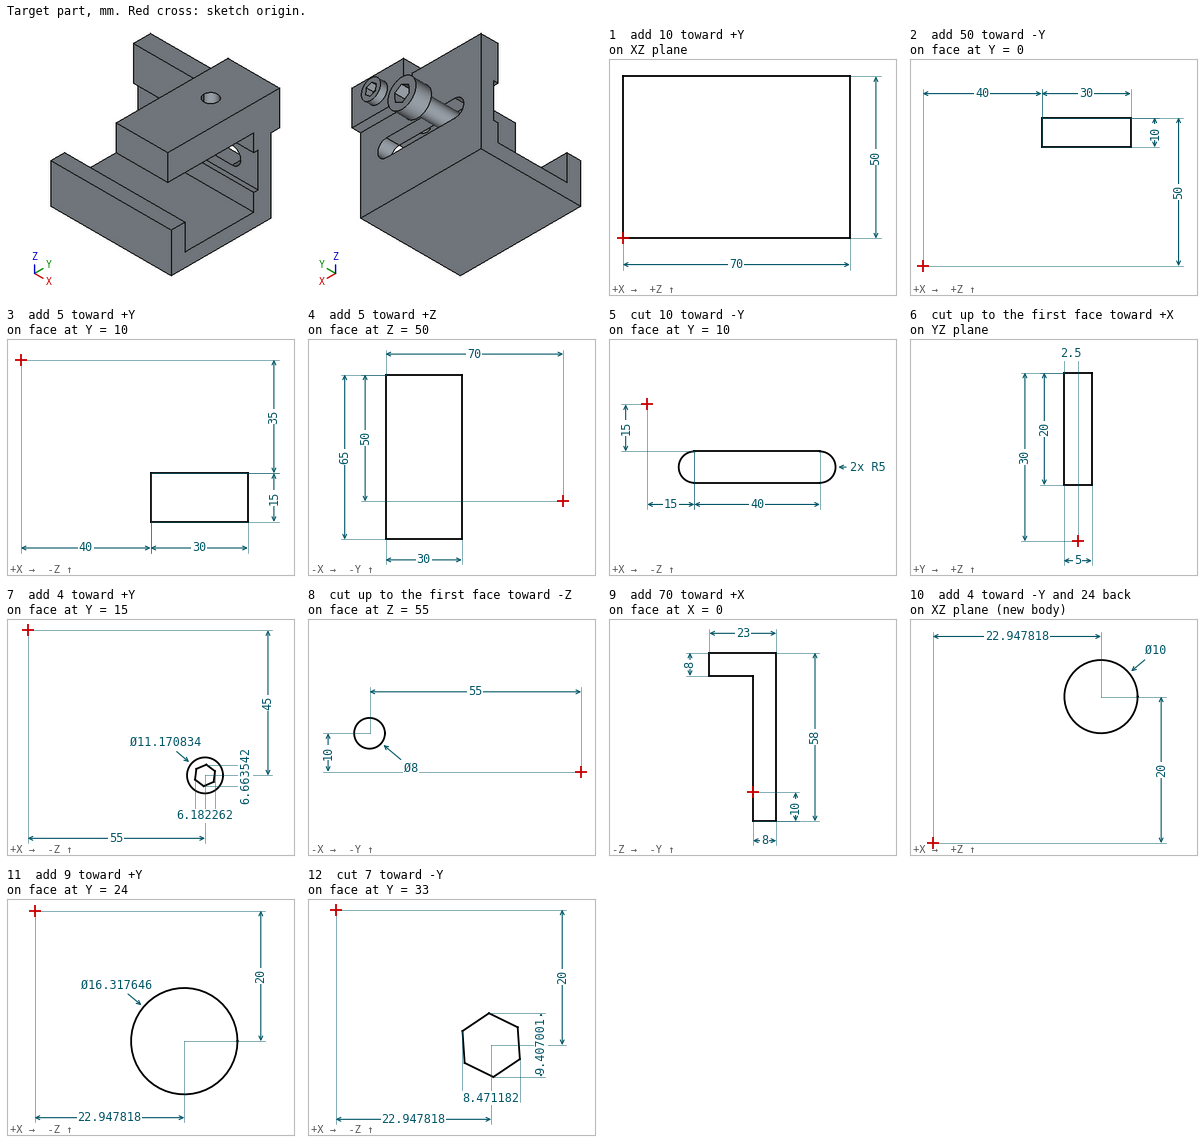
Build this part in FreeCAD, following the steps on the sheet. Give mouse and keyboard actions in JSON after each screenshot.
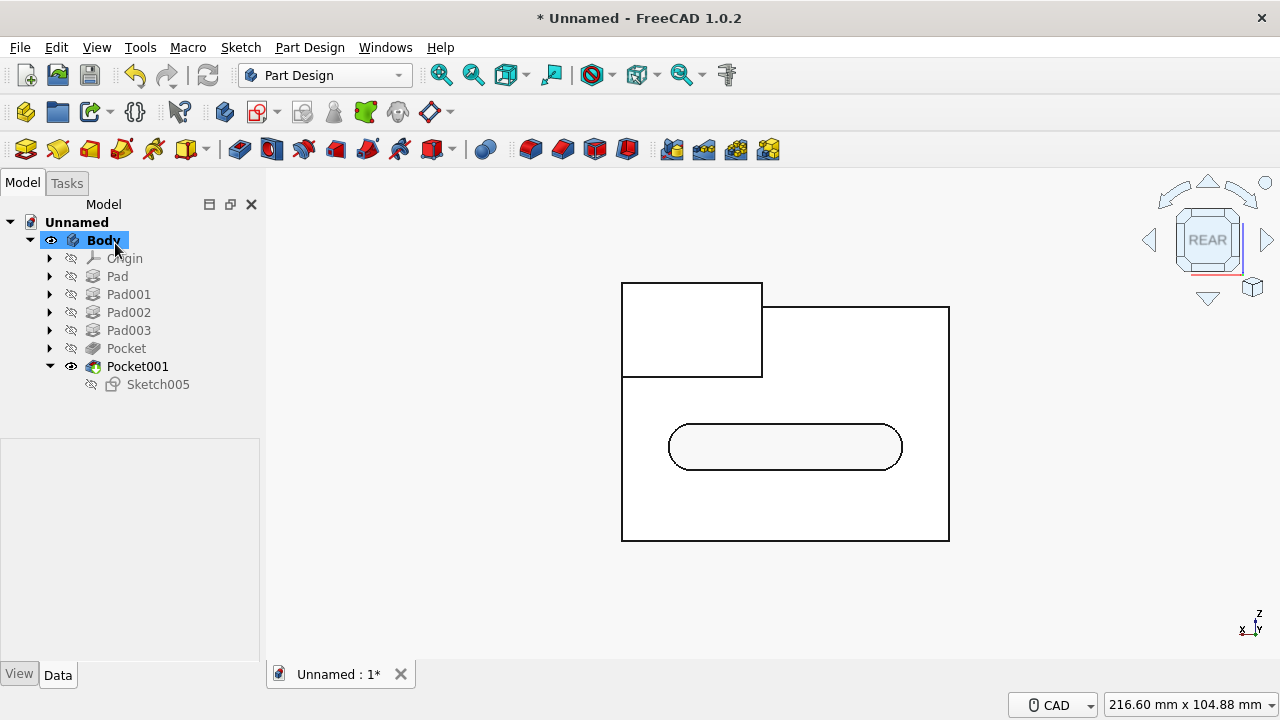
{"action": "left_click", "coordinate": [672, 329]}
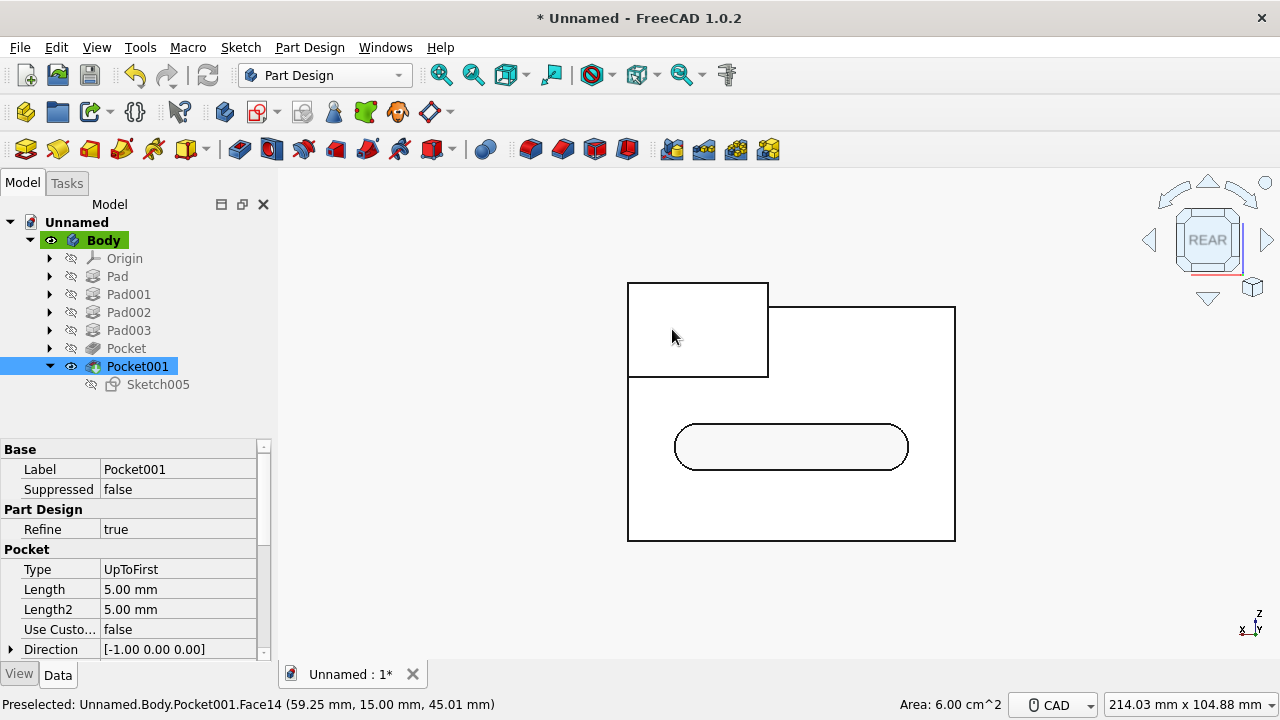
{"action": "left_click", "coordinate": [258, 112]}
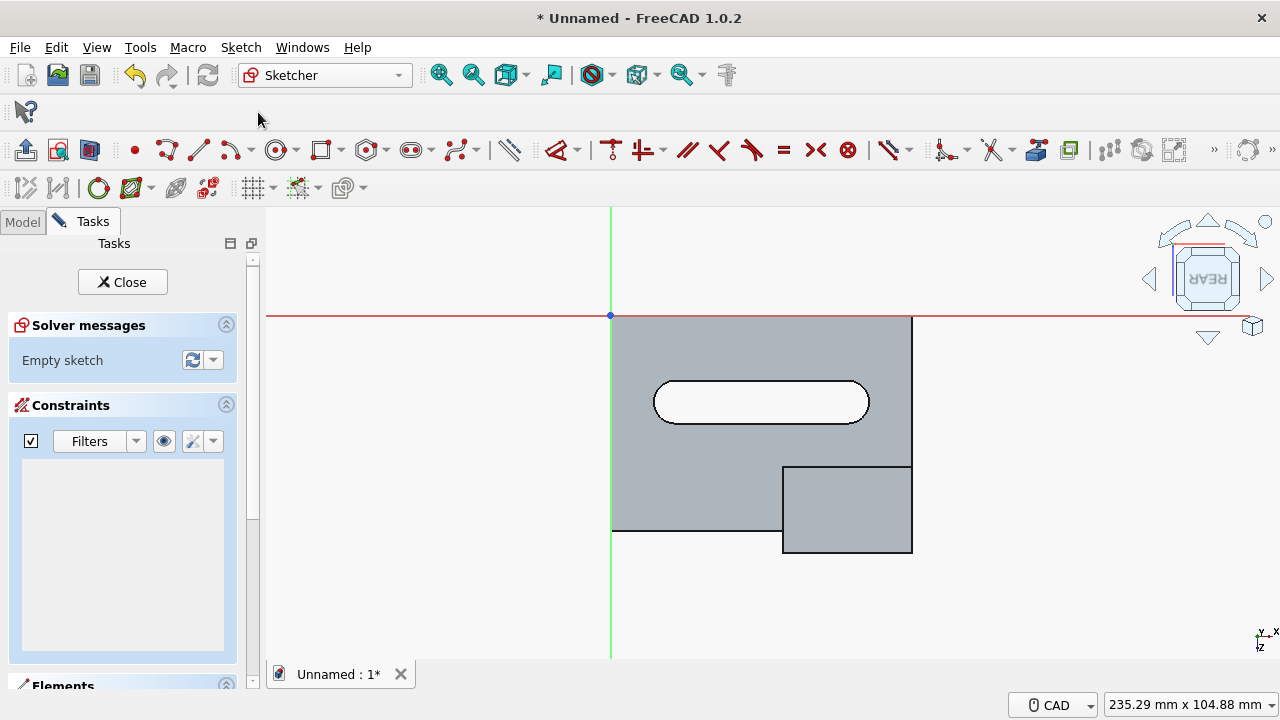
{"action": "scroll", "coordinate": [876, 525], "scroll_direction": "up", "scroll_amount": 9}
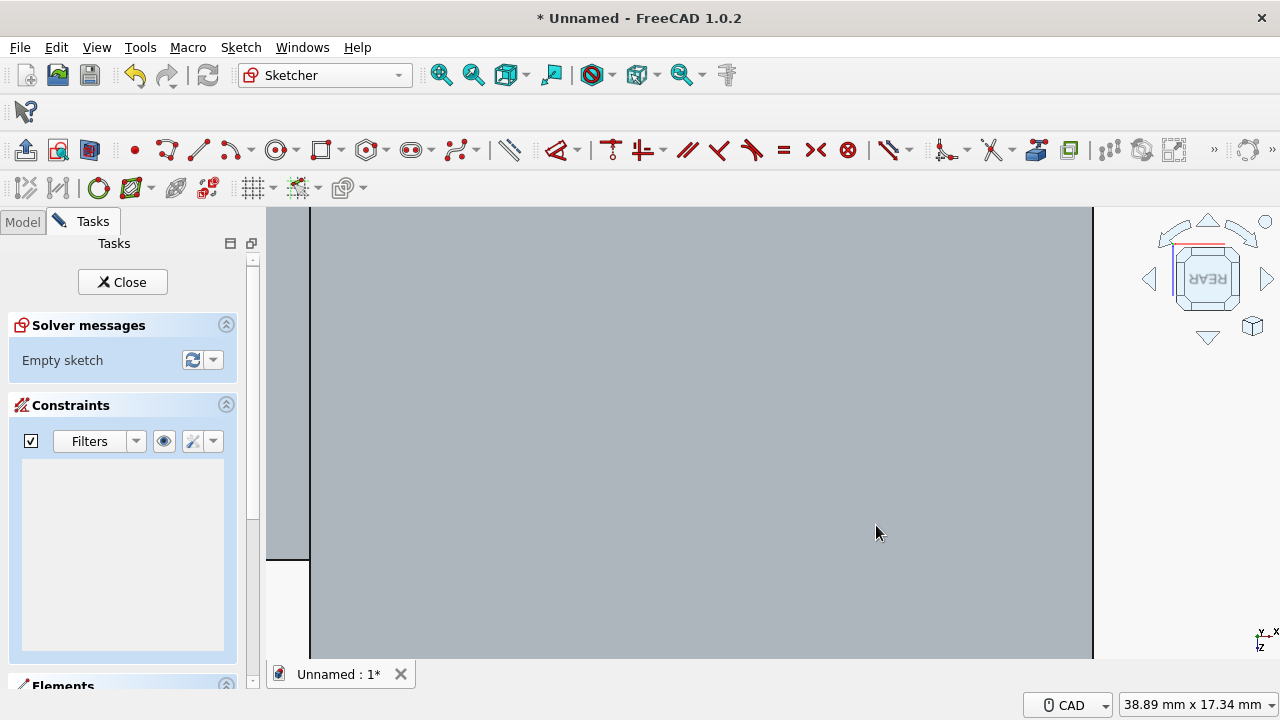
{"action": "left_click", "coordinate": [366, 150]}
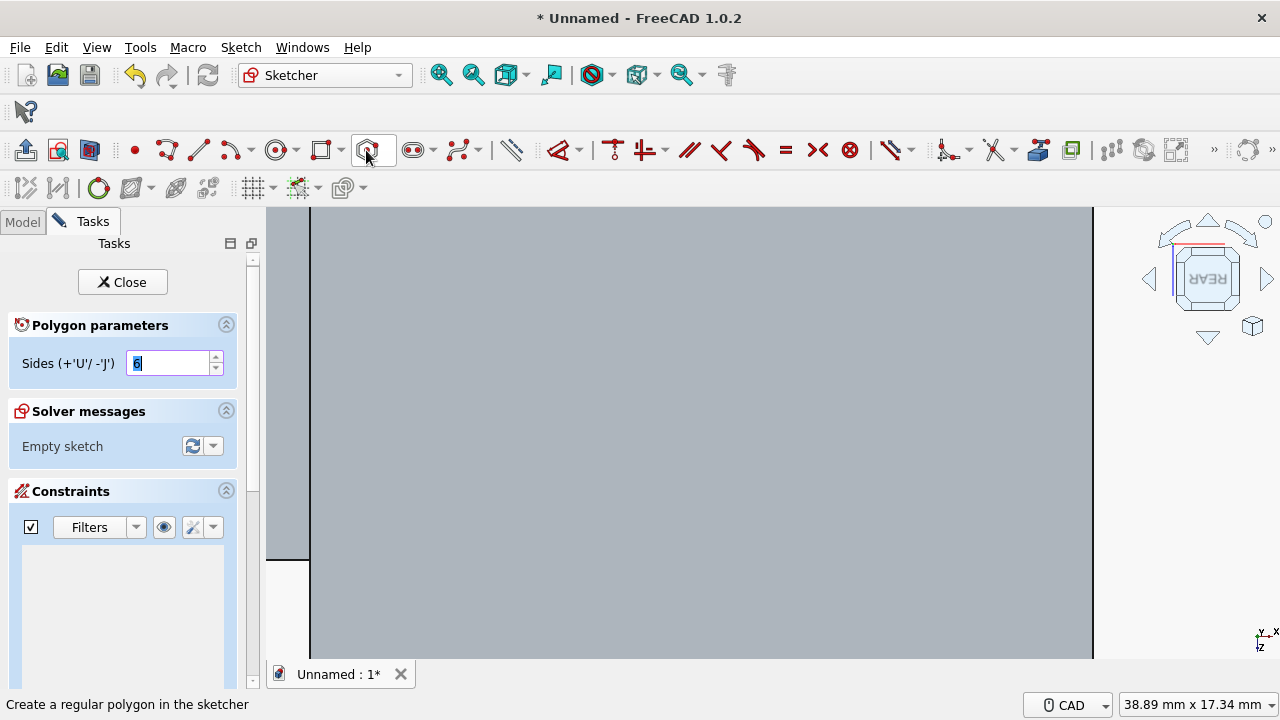
{"action": "left_click", "coordinate": [702, 430]}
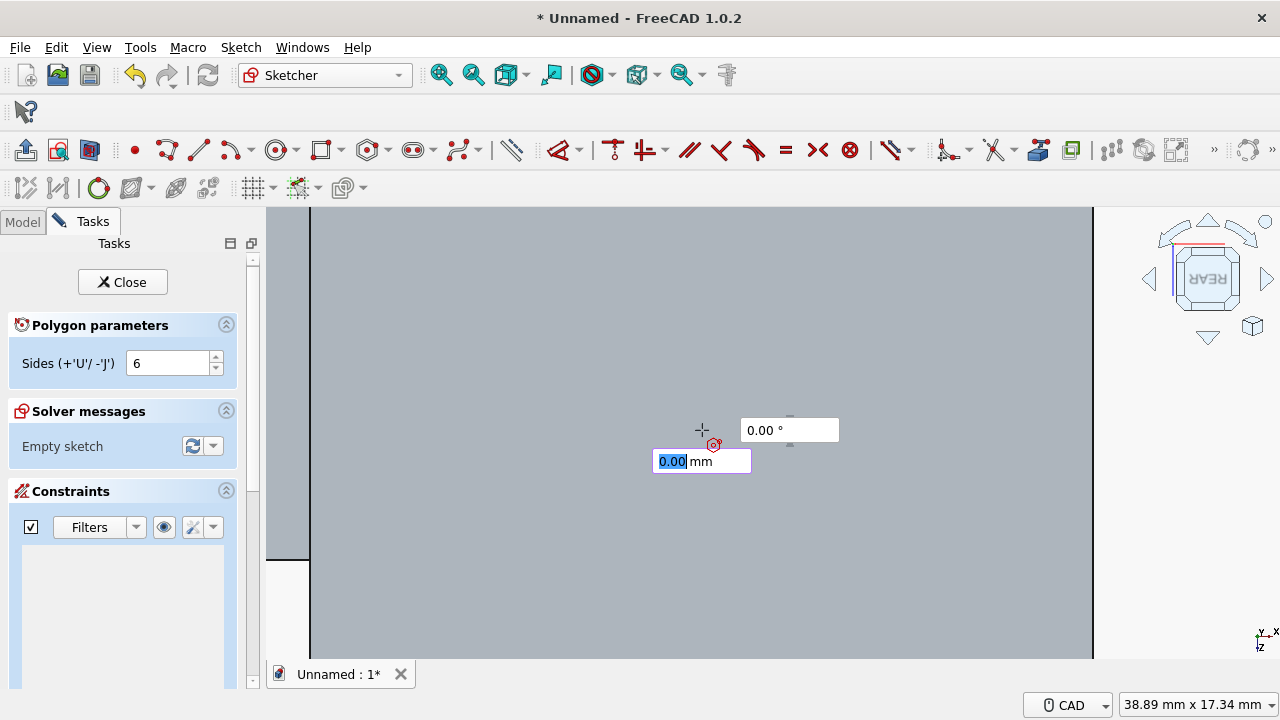
{"action": "left_click", "coordinate": [691, 517]}
{"action": "key", "text": "Escape"}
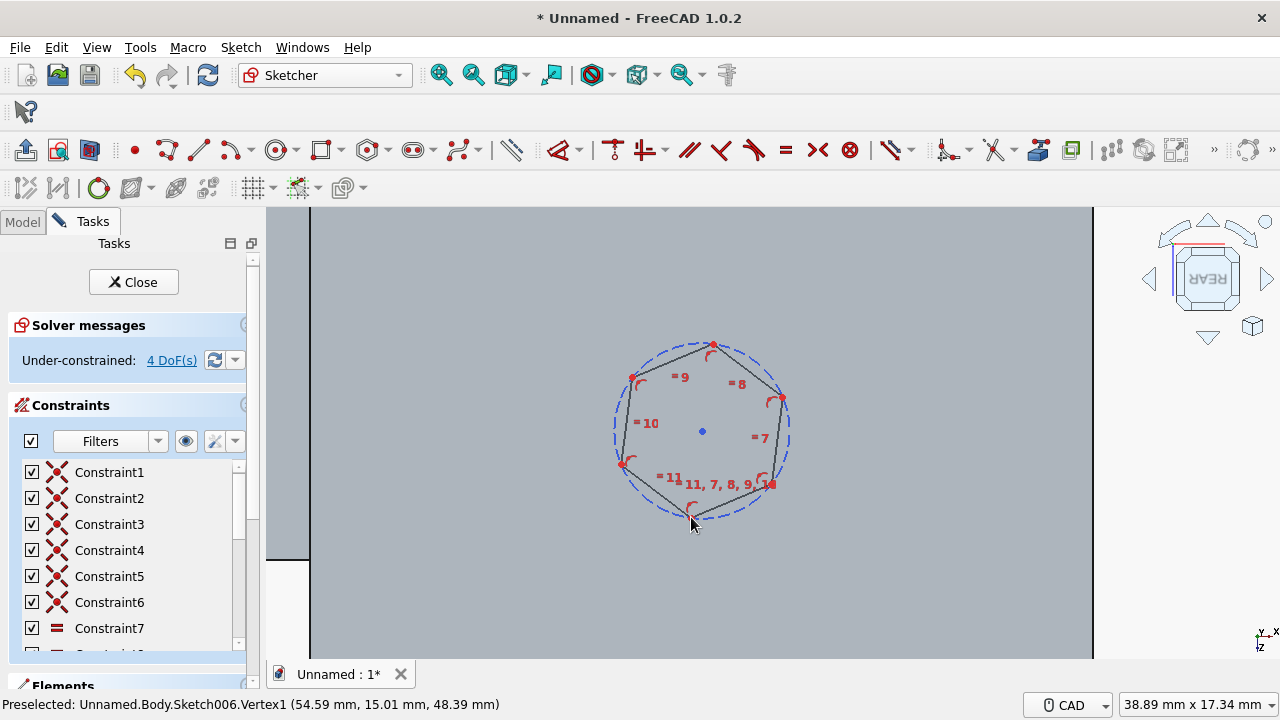
{"action": "left_click", "coordinate": [276, 150]}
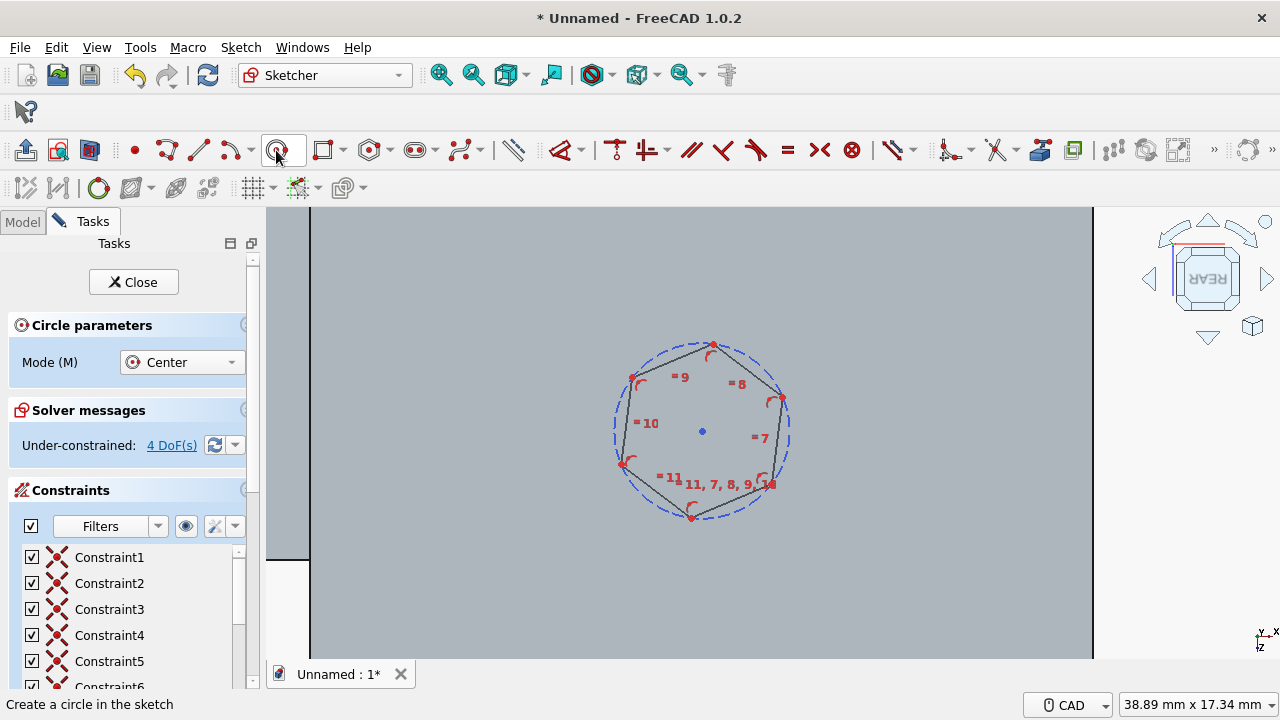
{"action": "left_click", "coordinate": [702, 431]}
{"action": "left_click", "coordinate": [805, 327]}
{"action": "key", "text": "Escape"}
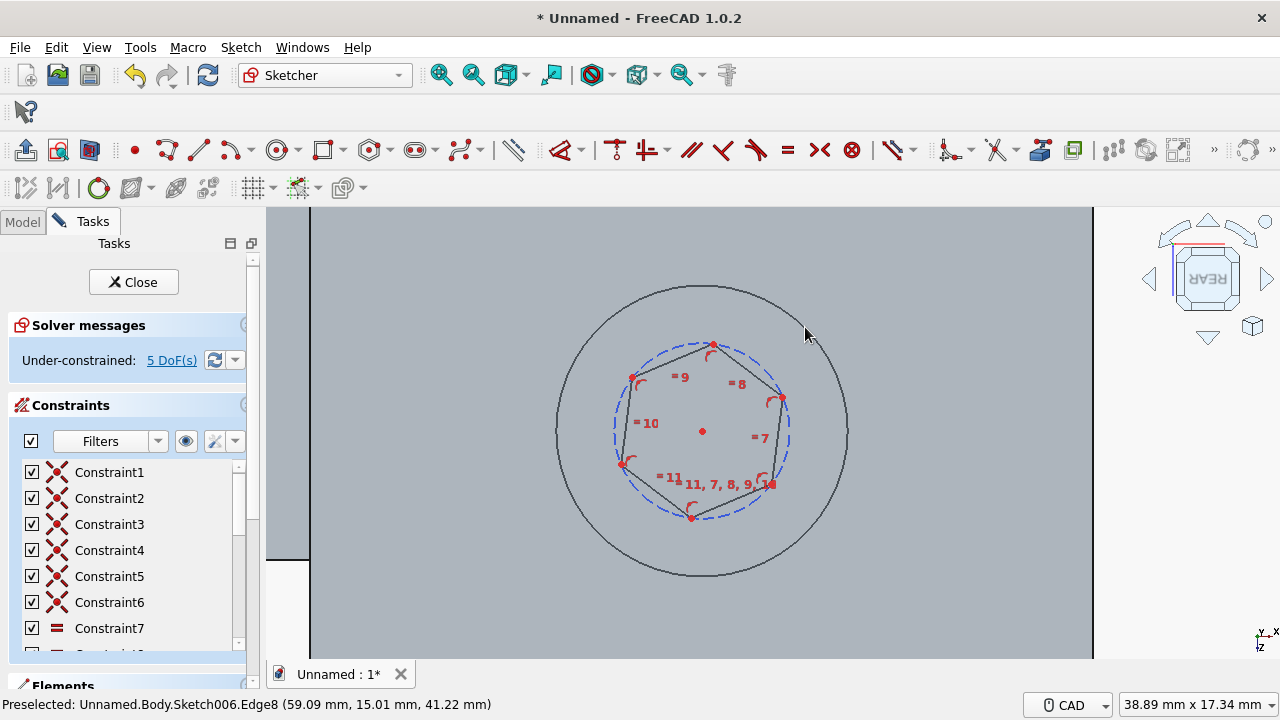
{"action": "left_click", "coordinate": [560, 150]}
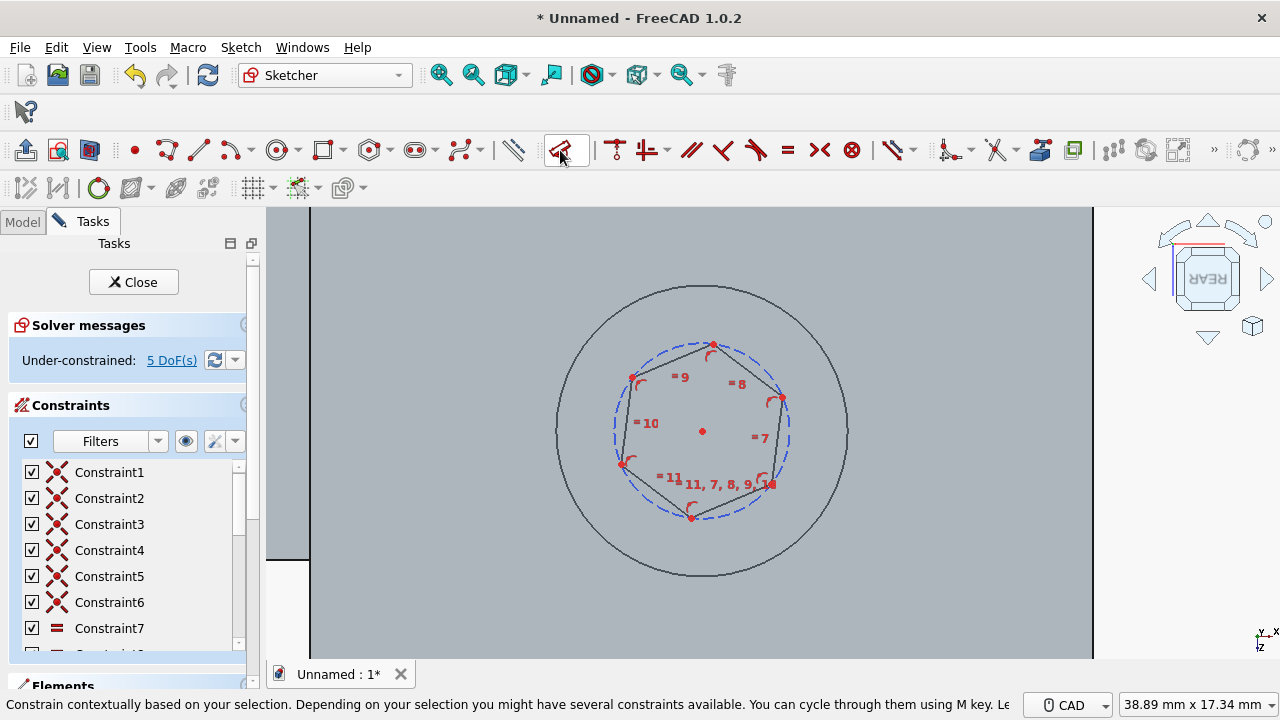
{"action": "left_click", "coordinate": [805, 328]}
{"action": "left_click", "coordinate": [828, 305]}